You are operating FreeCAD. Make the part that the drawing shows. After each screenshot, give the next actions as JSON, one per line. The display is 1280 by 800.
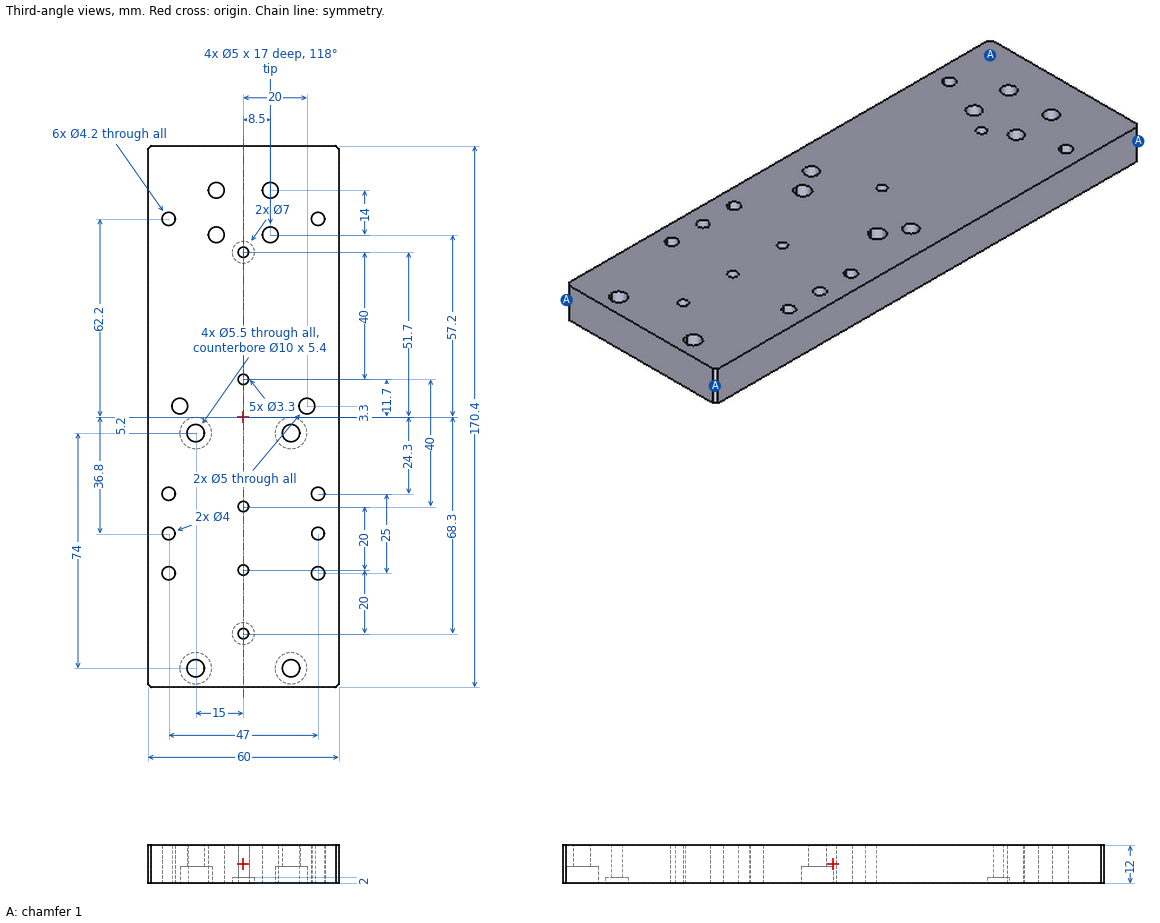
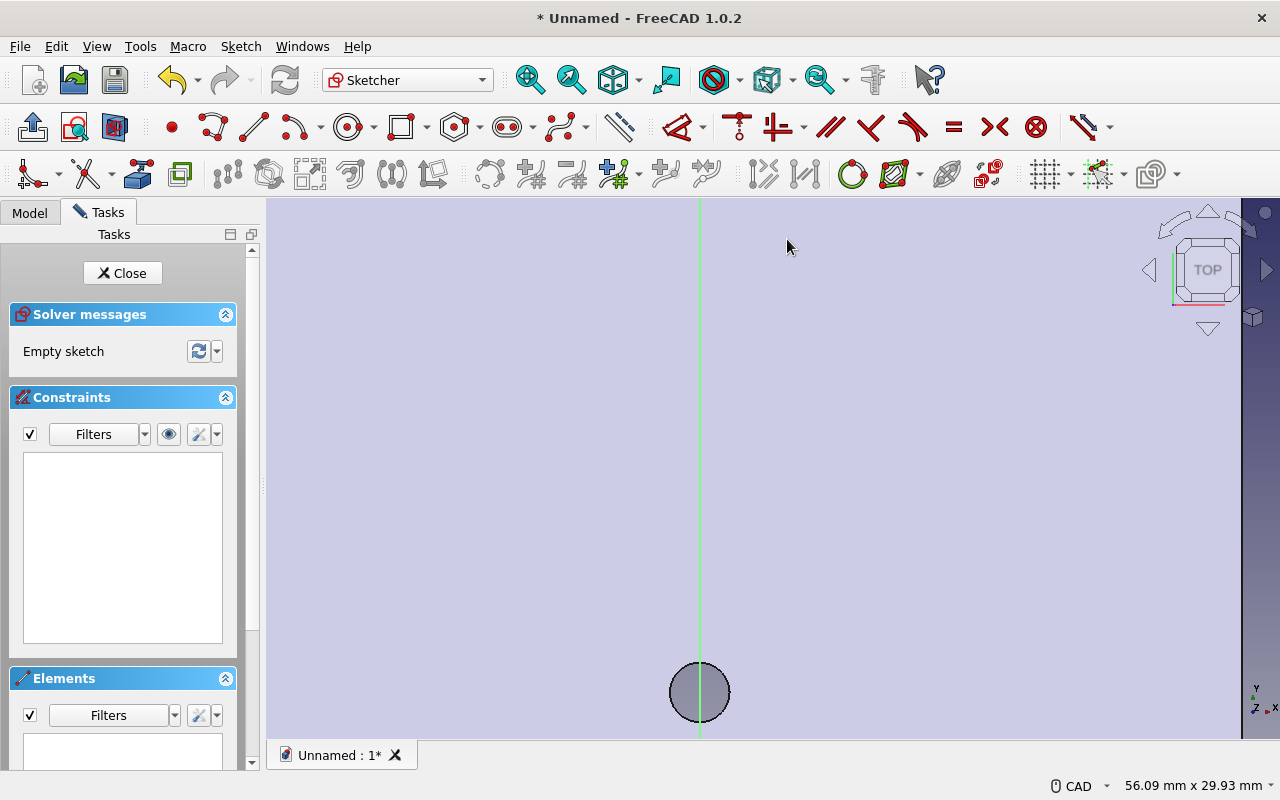
{"action": "left_click", "coordinate": [348, 128]}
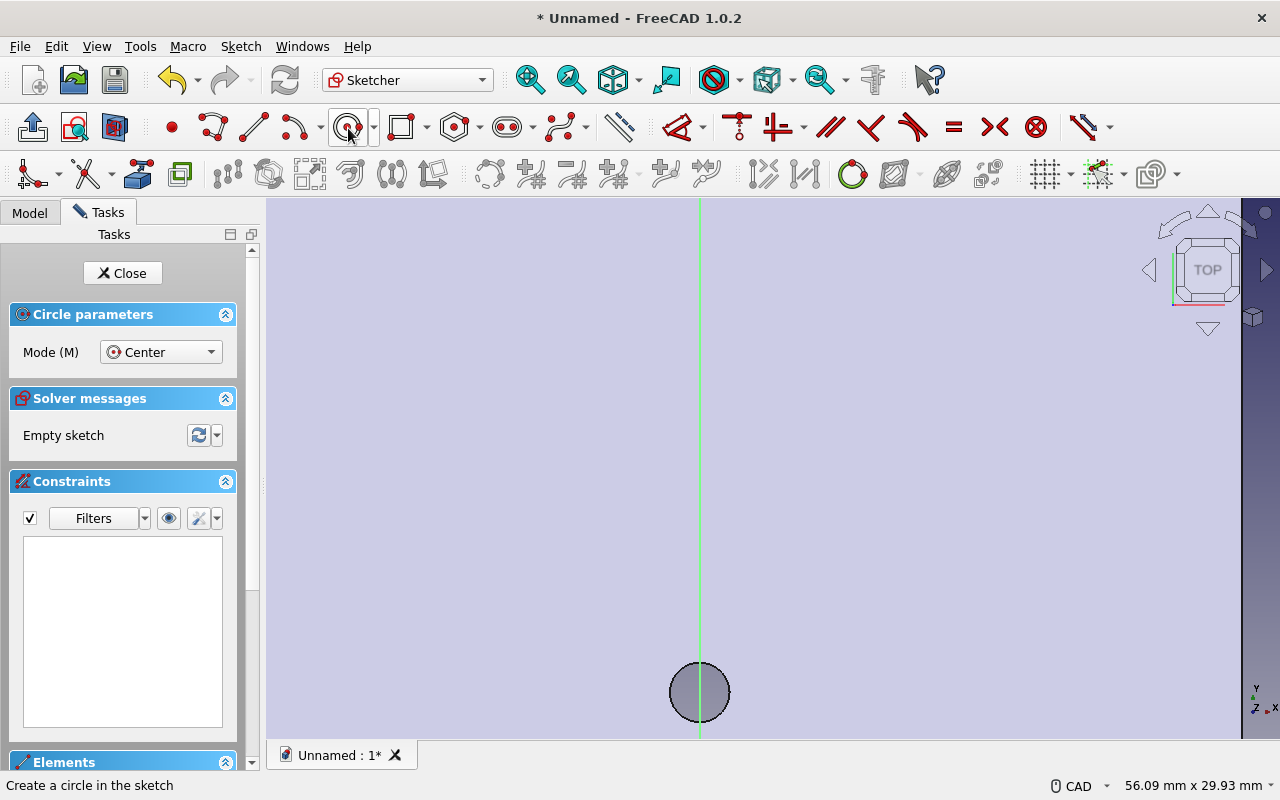
{"action": "left_click", "coordinate": [853, 593]}
{"action": "left_click", "coordinate": [885, 561]}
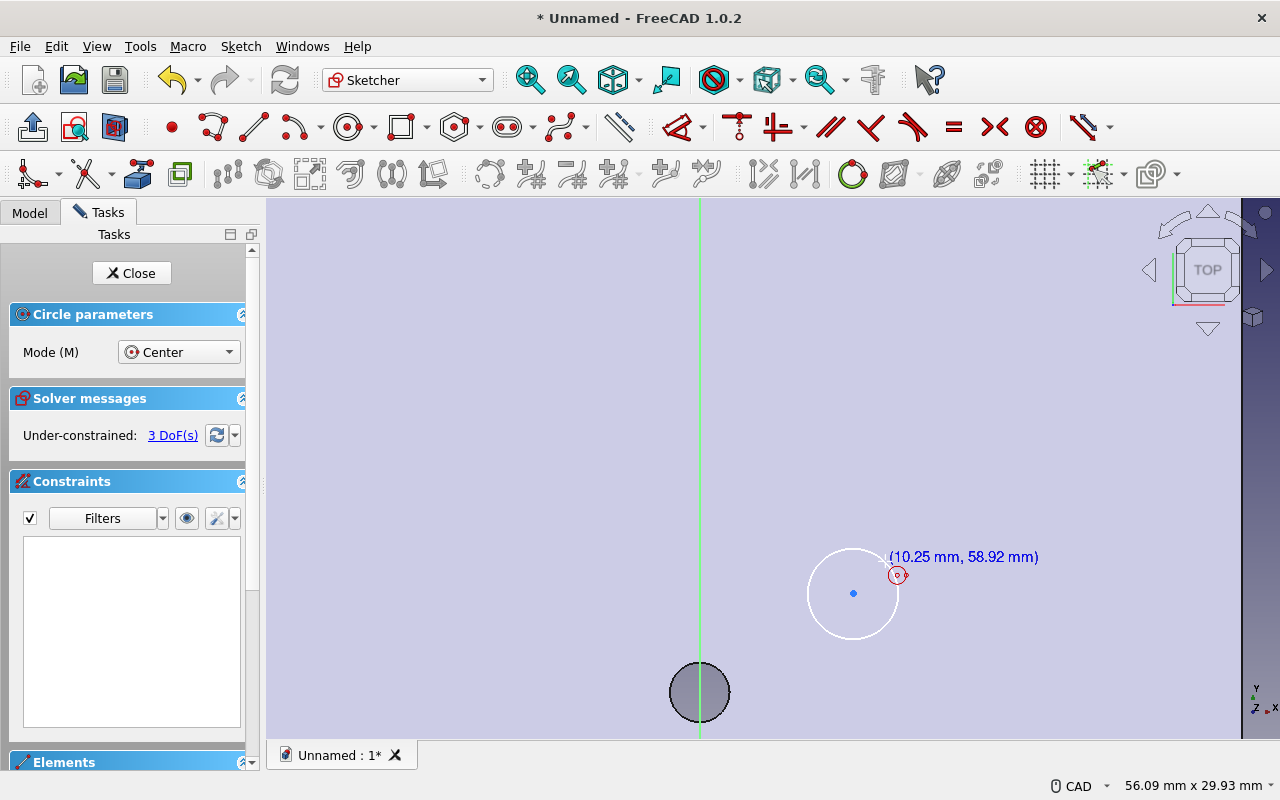
{"action": "left_click", "coordinate": [546, 593]}
{"action": "left_click", "coordinate": [578, 561]}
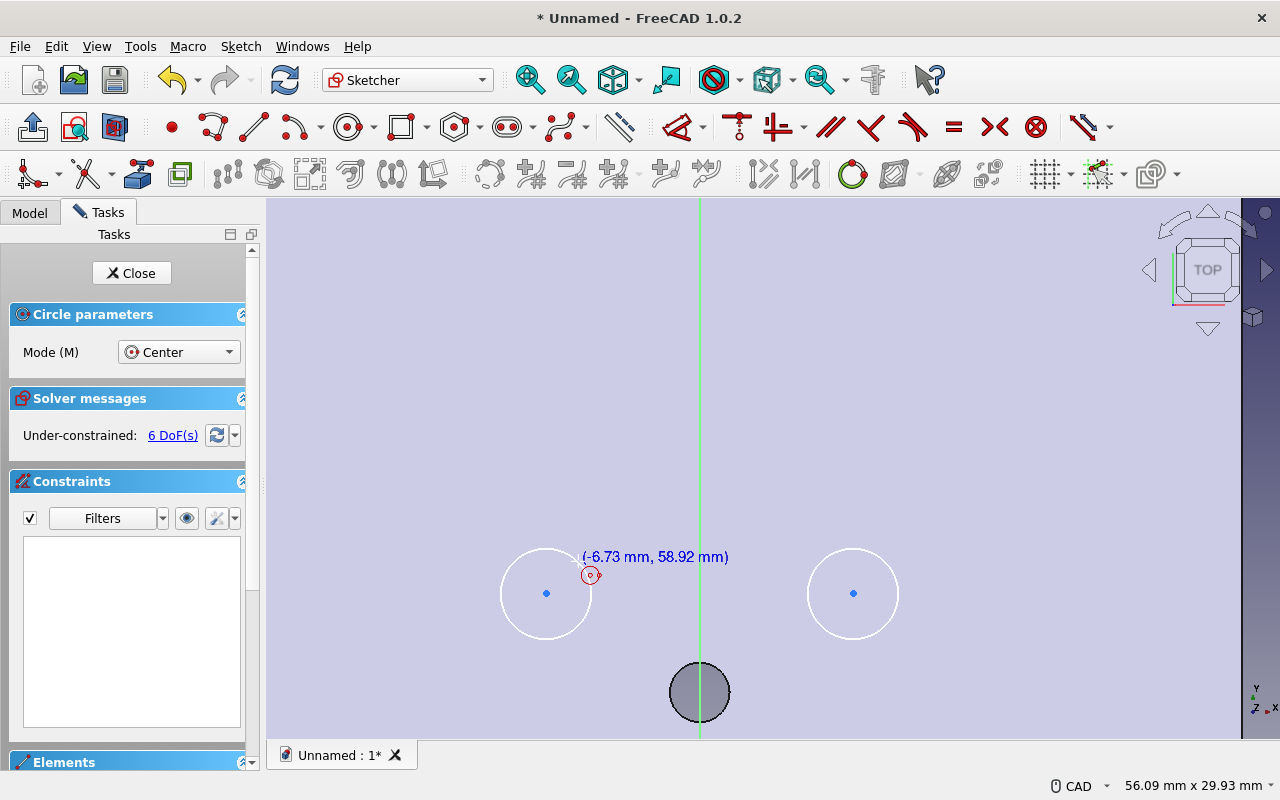
{"action": "left_click", "coordinate": [853, 340]}
{"action": "left_click", "coordinate": [885, 308]}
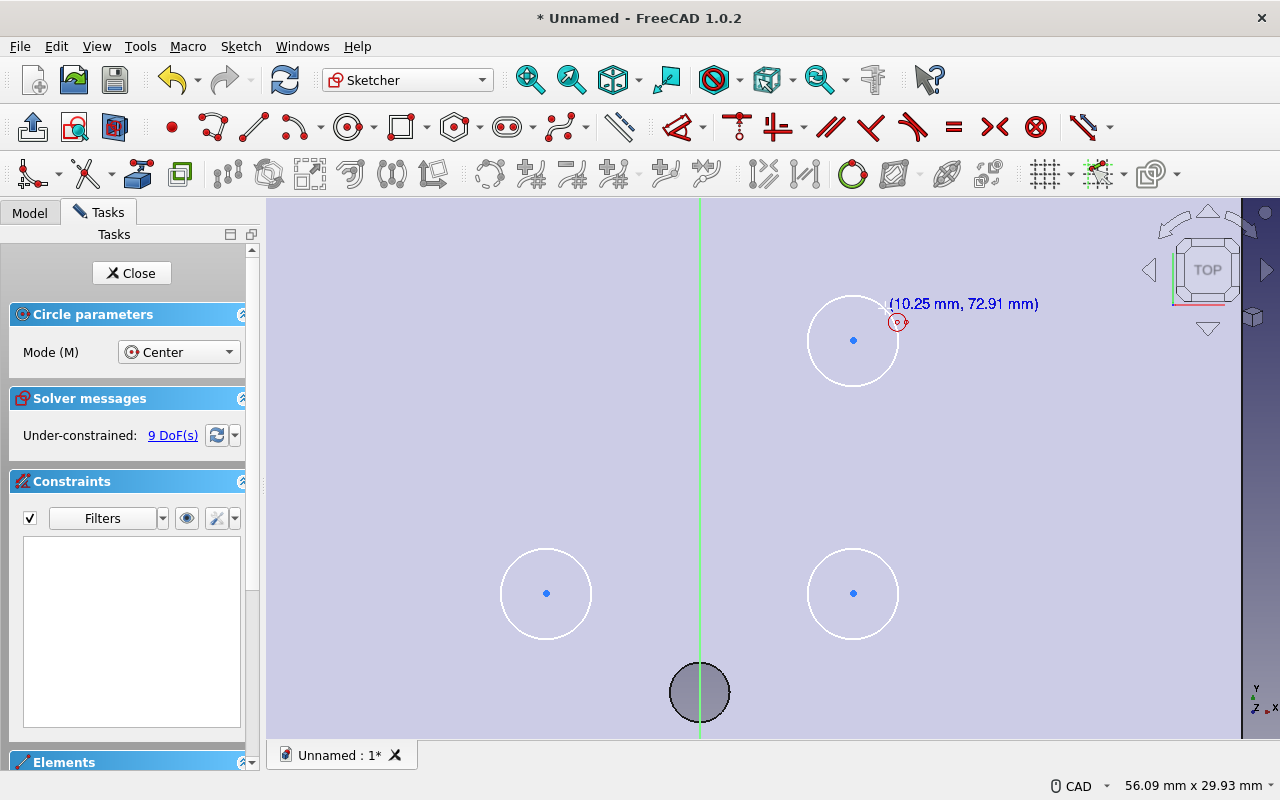
{"action": "left_click", "coordinate": [546, 340]}
{"action": "left_click", "coordinate": [578, 308]}
{"action": "key", "text": "Escape"}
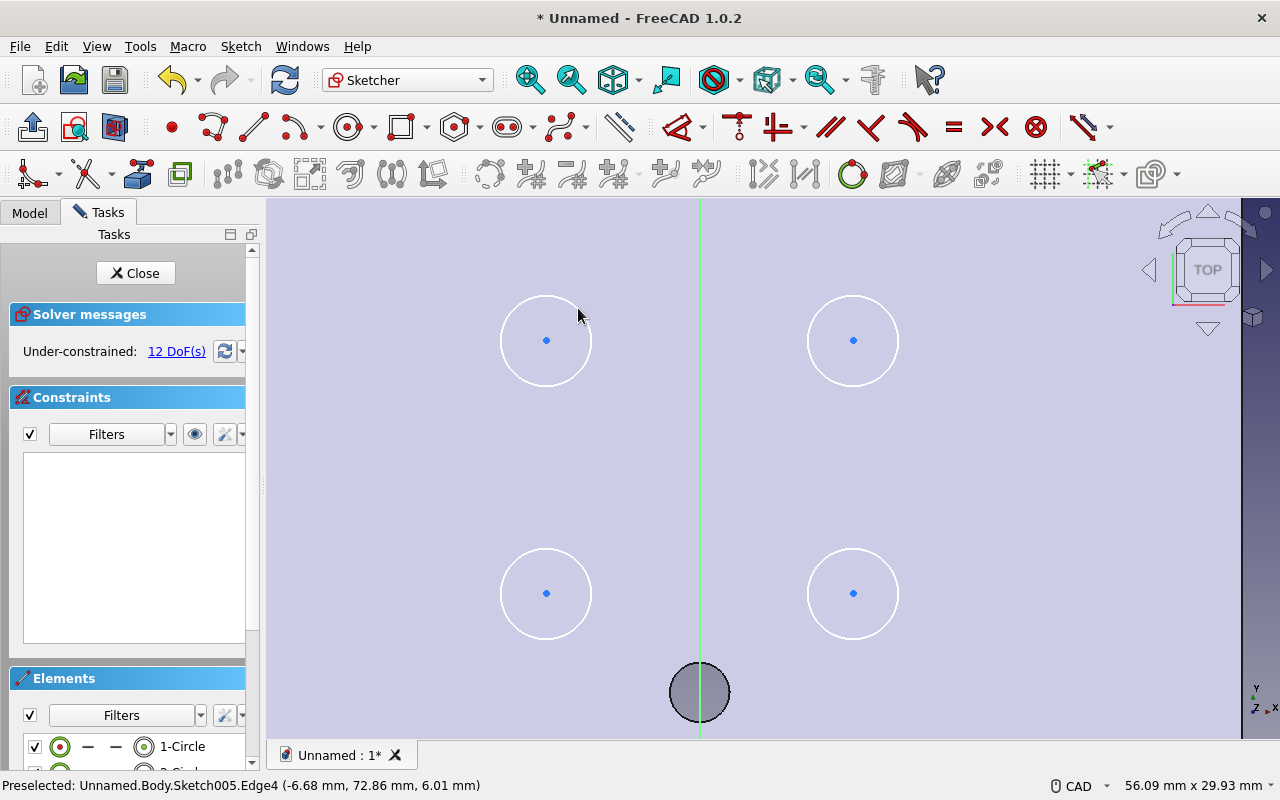
{"action": "left_click", "coordinate": [885, 562]}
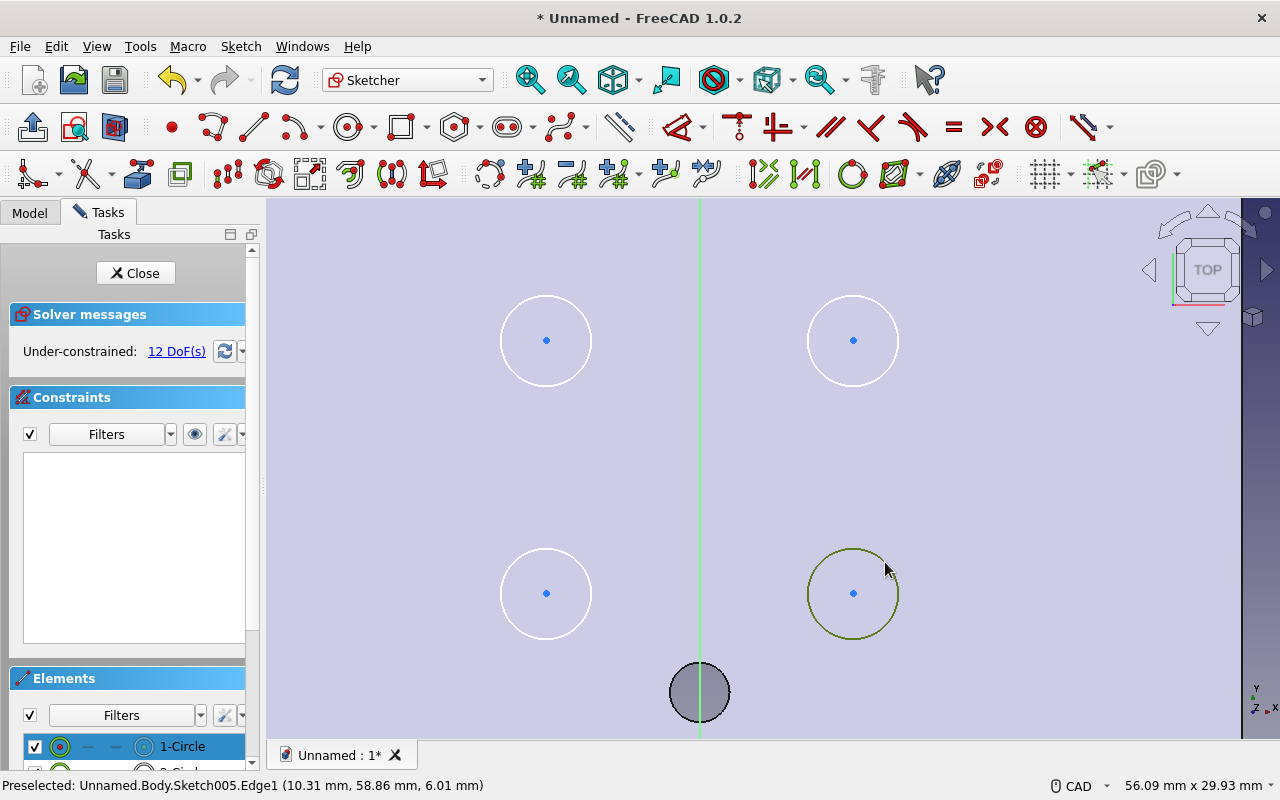
{"action": "left_click", "coordinate": [578, 562]}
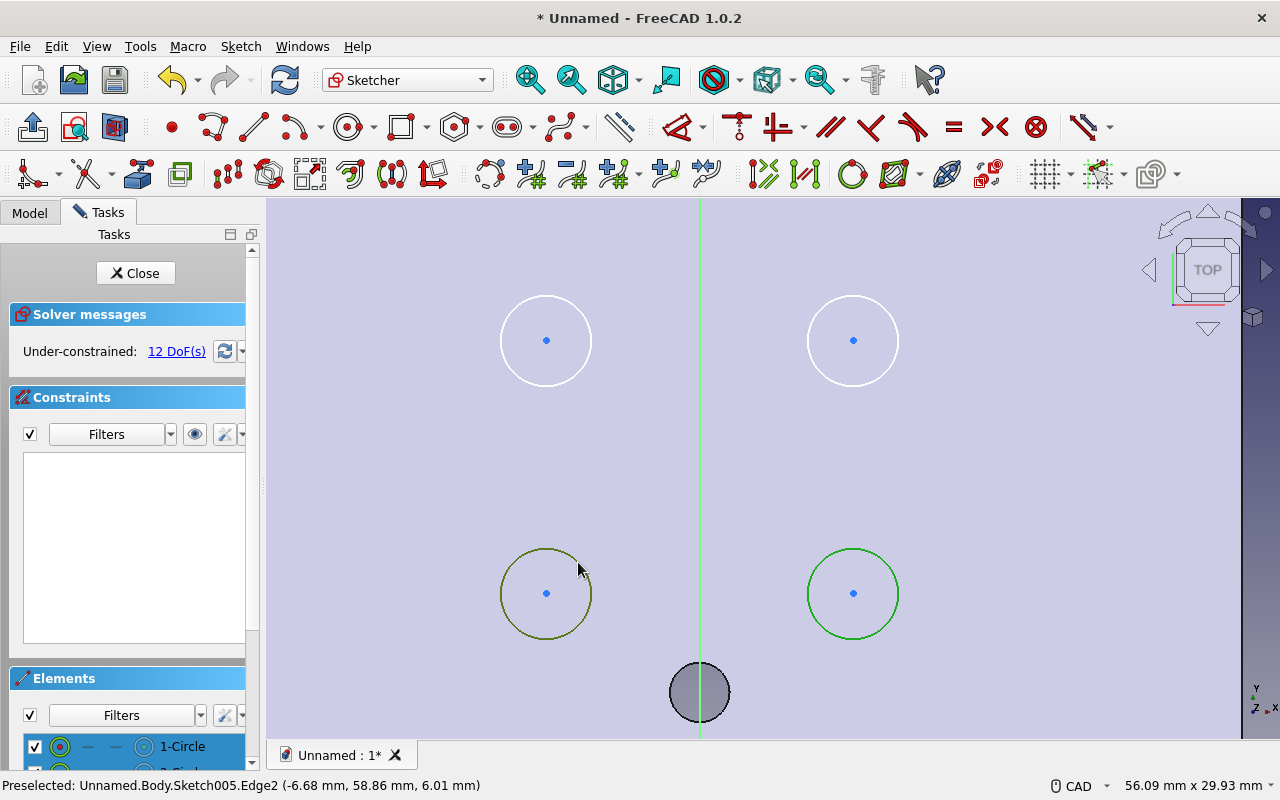
{"action": "left_click", "coordinate": [885, 309]}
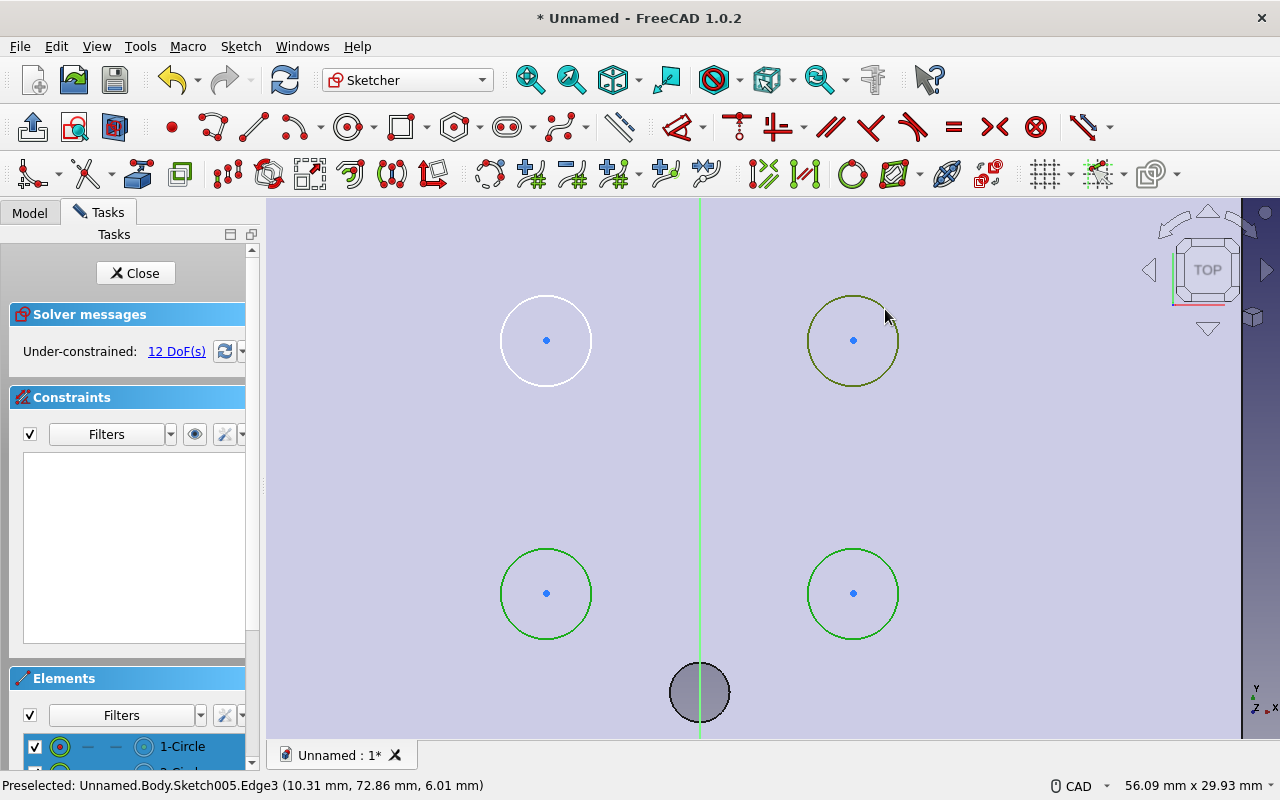
{"action": "left_click", "coordinate": [578, 309]}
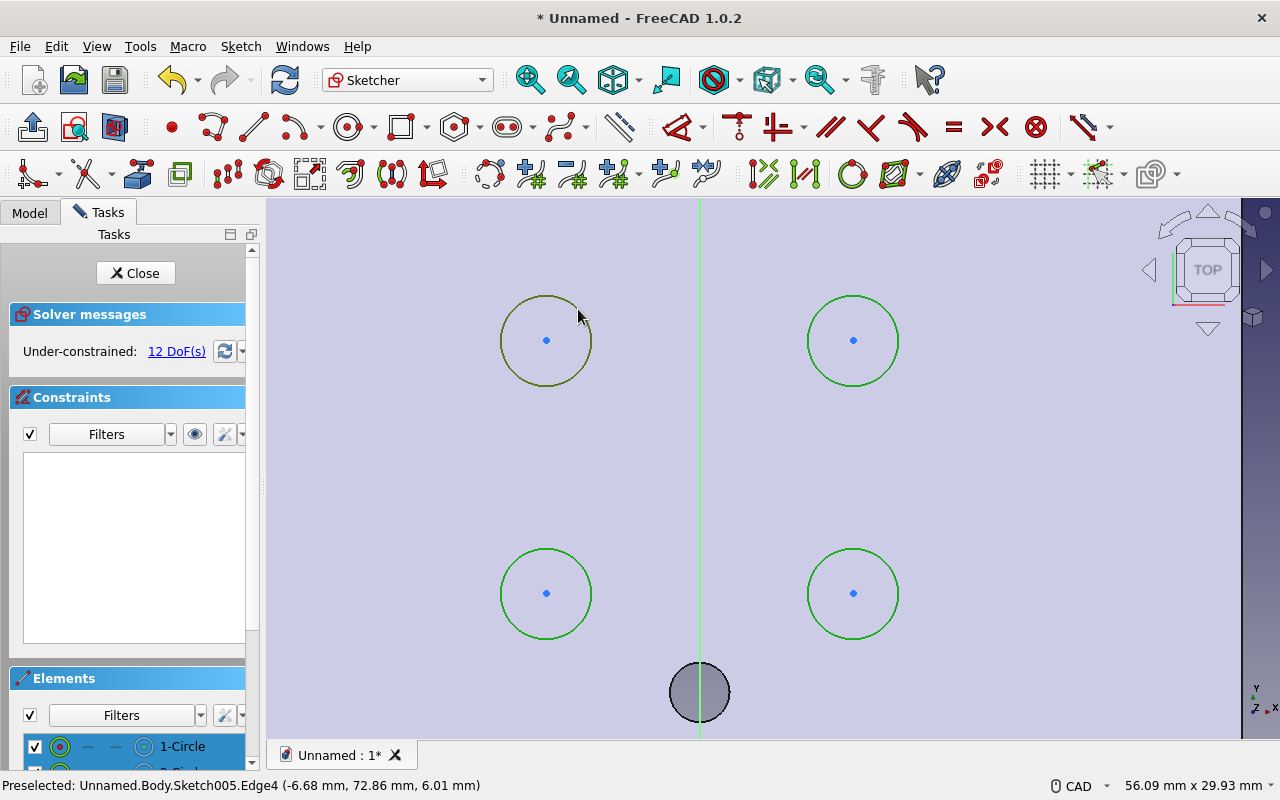
{"action": "left_click", "coordinate": [954, 128]}